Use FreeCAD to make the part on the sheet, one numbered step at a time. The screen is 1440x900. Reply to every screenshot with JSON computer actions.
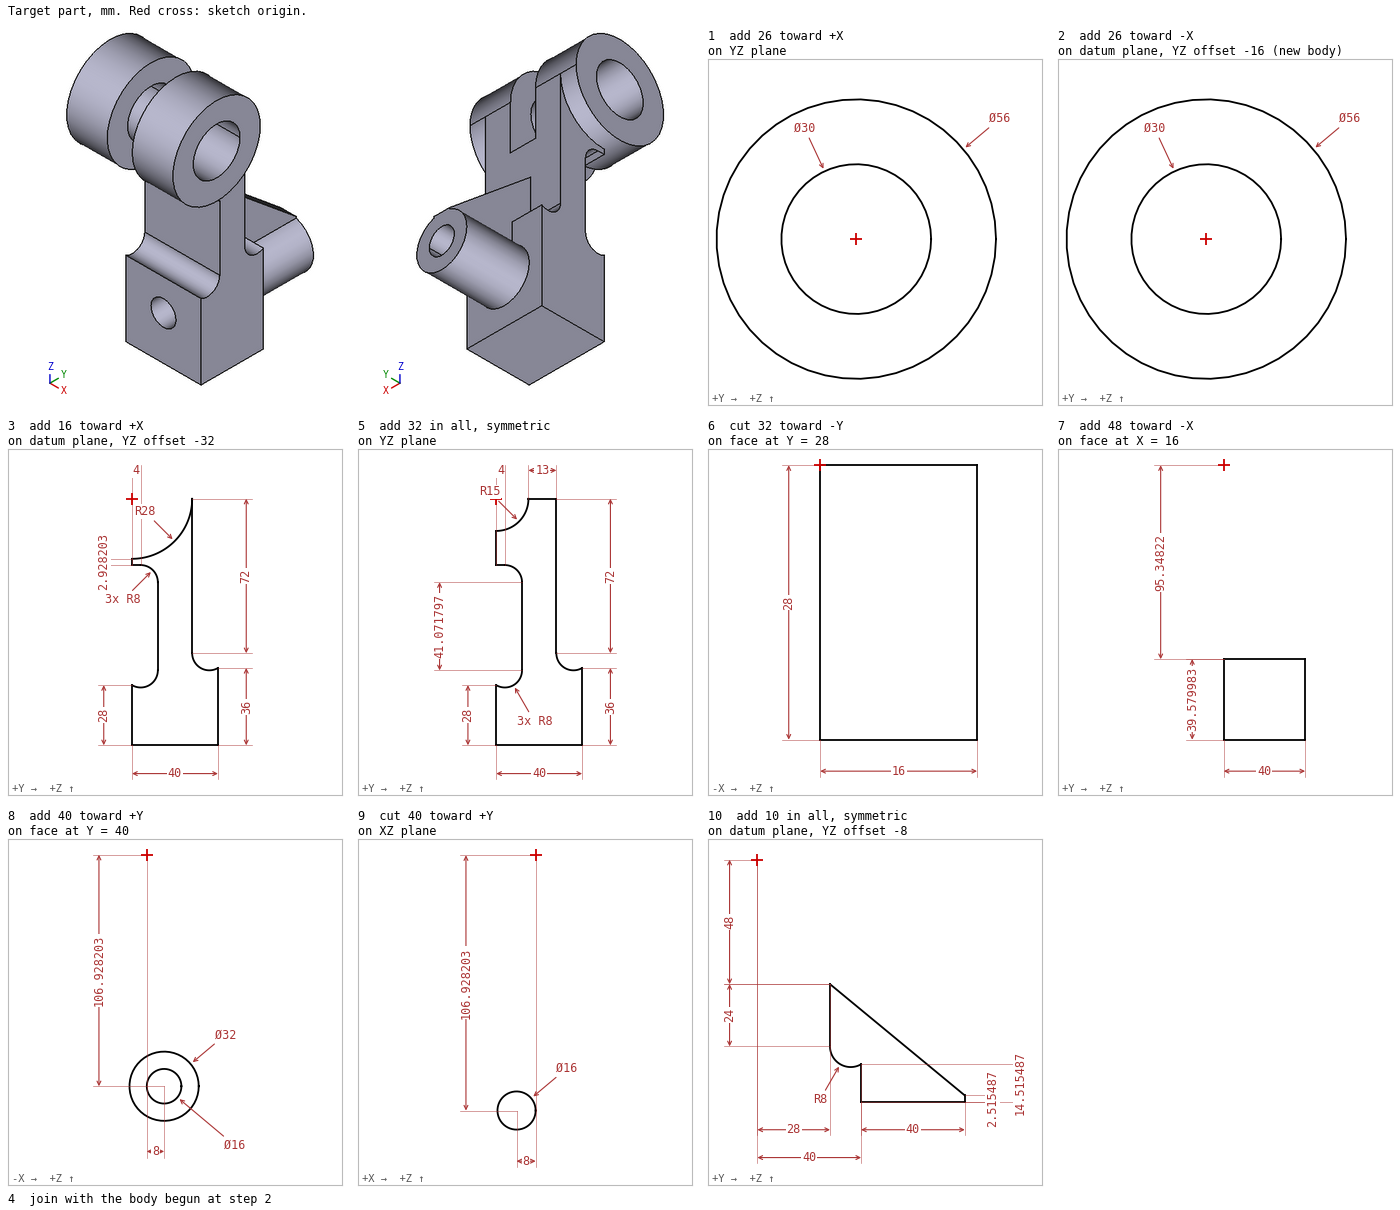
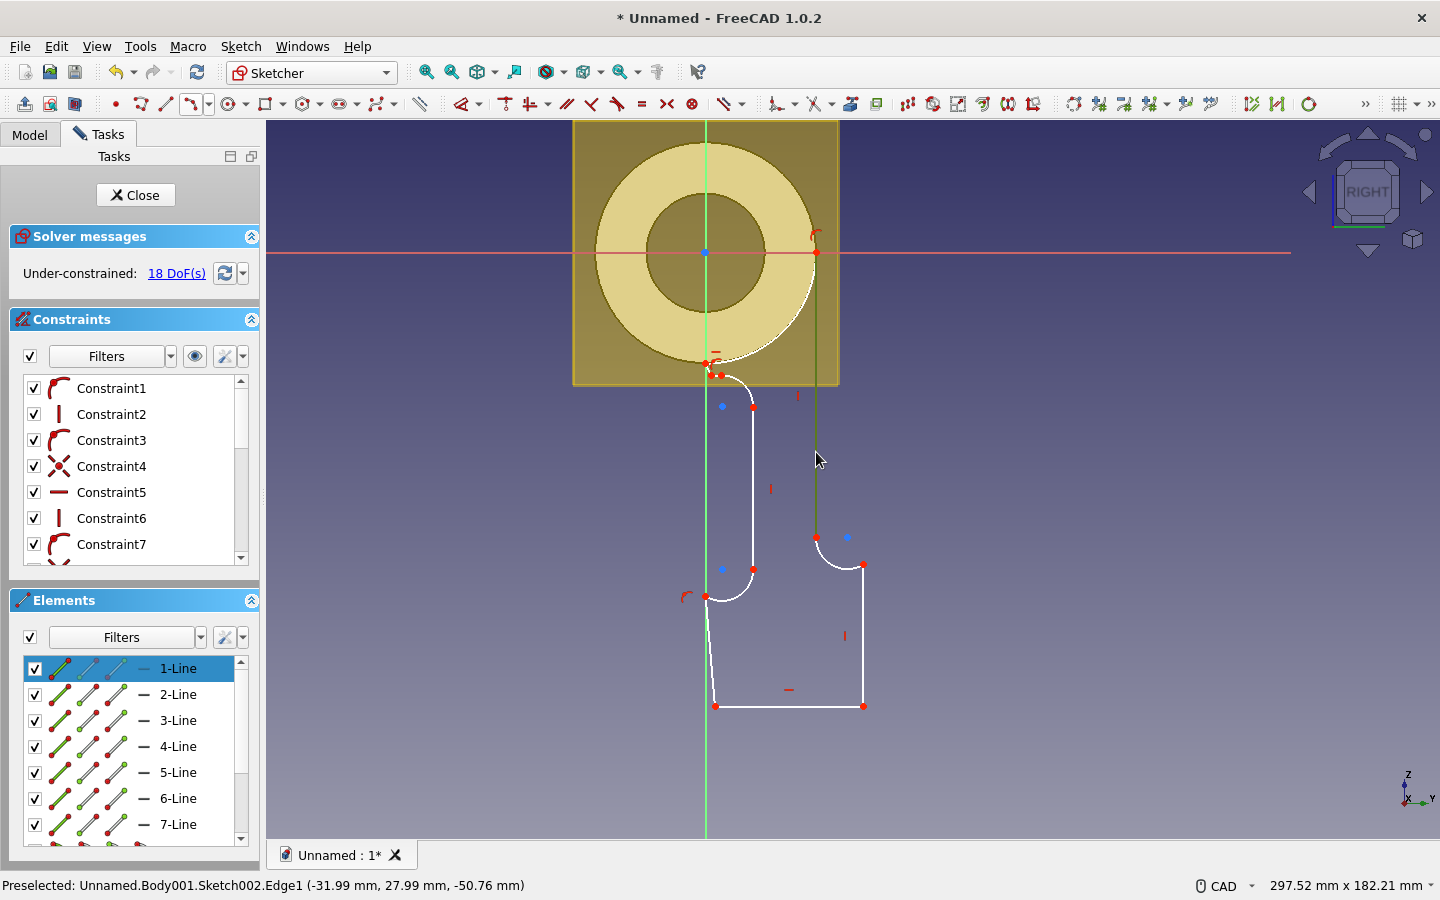
{"action": "left_click", "coordinate": [756, 351]}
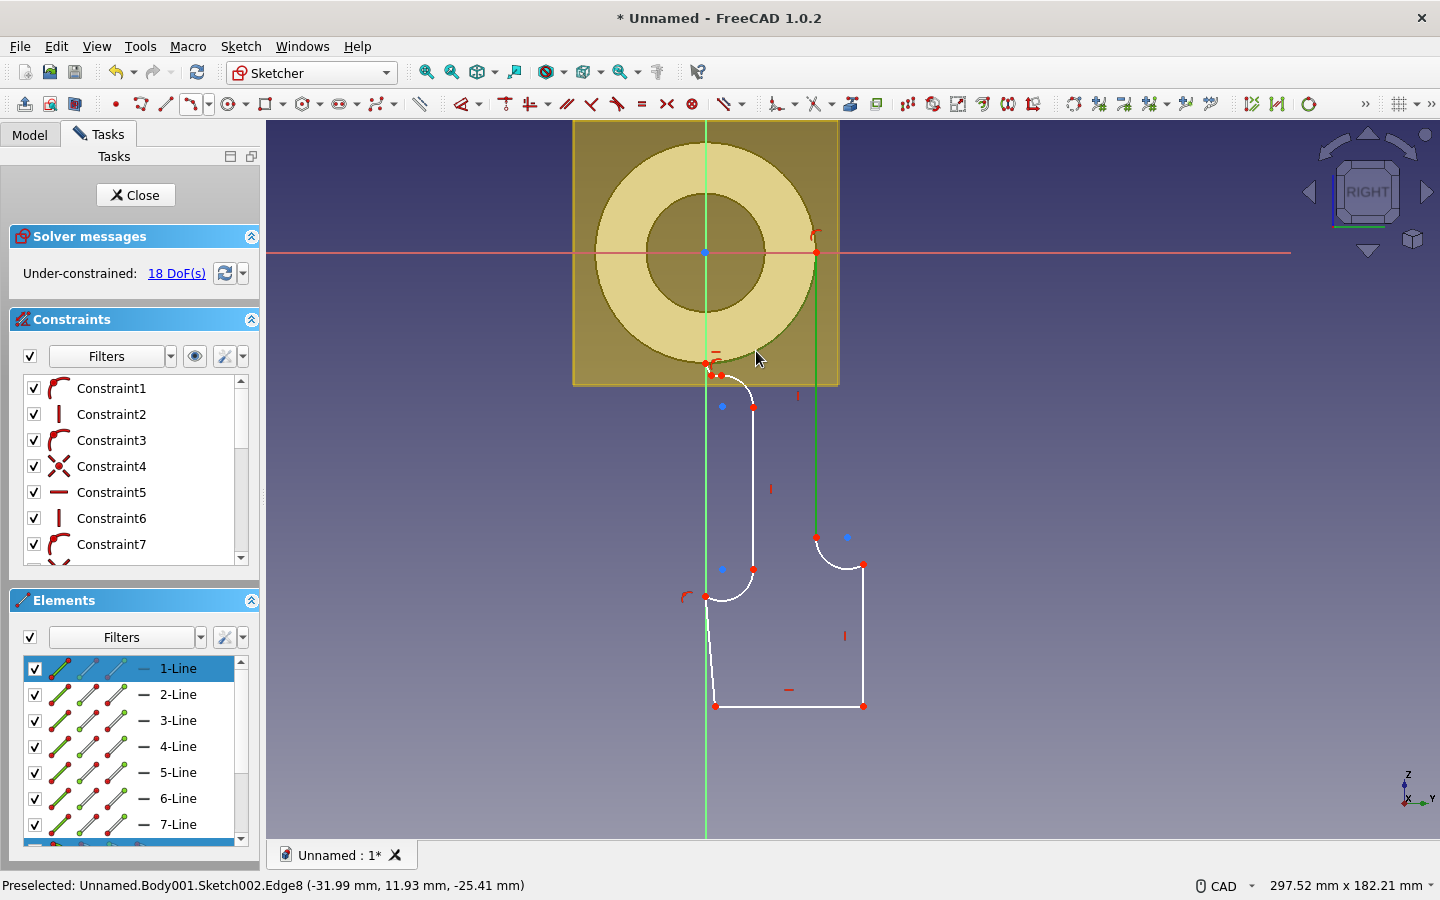
{"action": "key", "text": "t"}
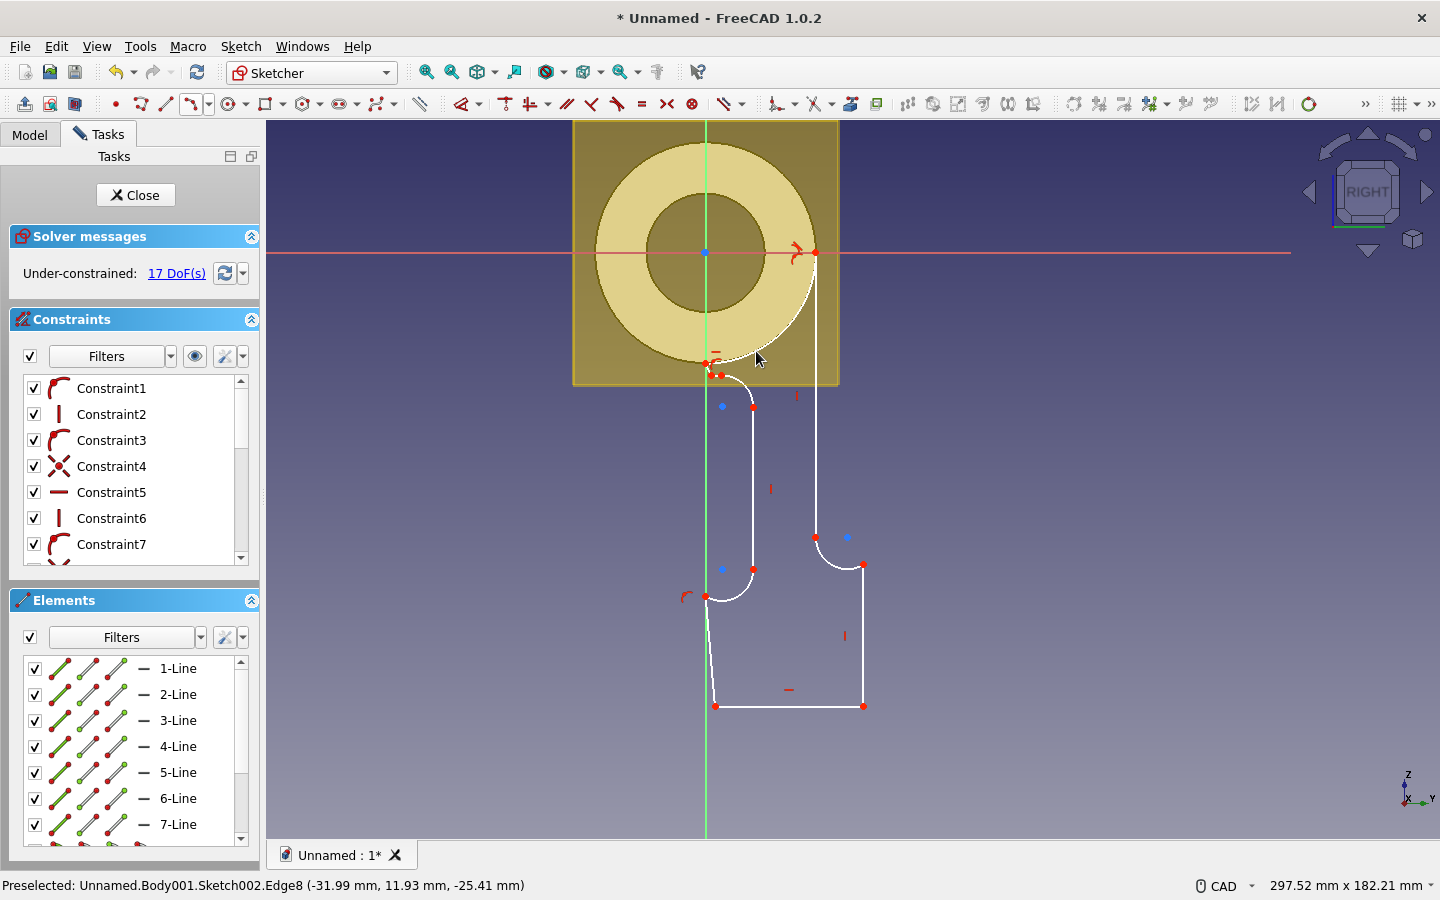
{"action": "left_click", "coordinate": [816, 452]}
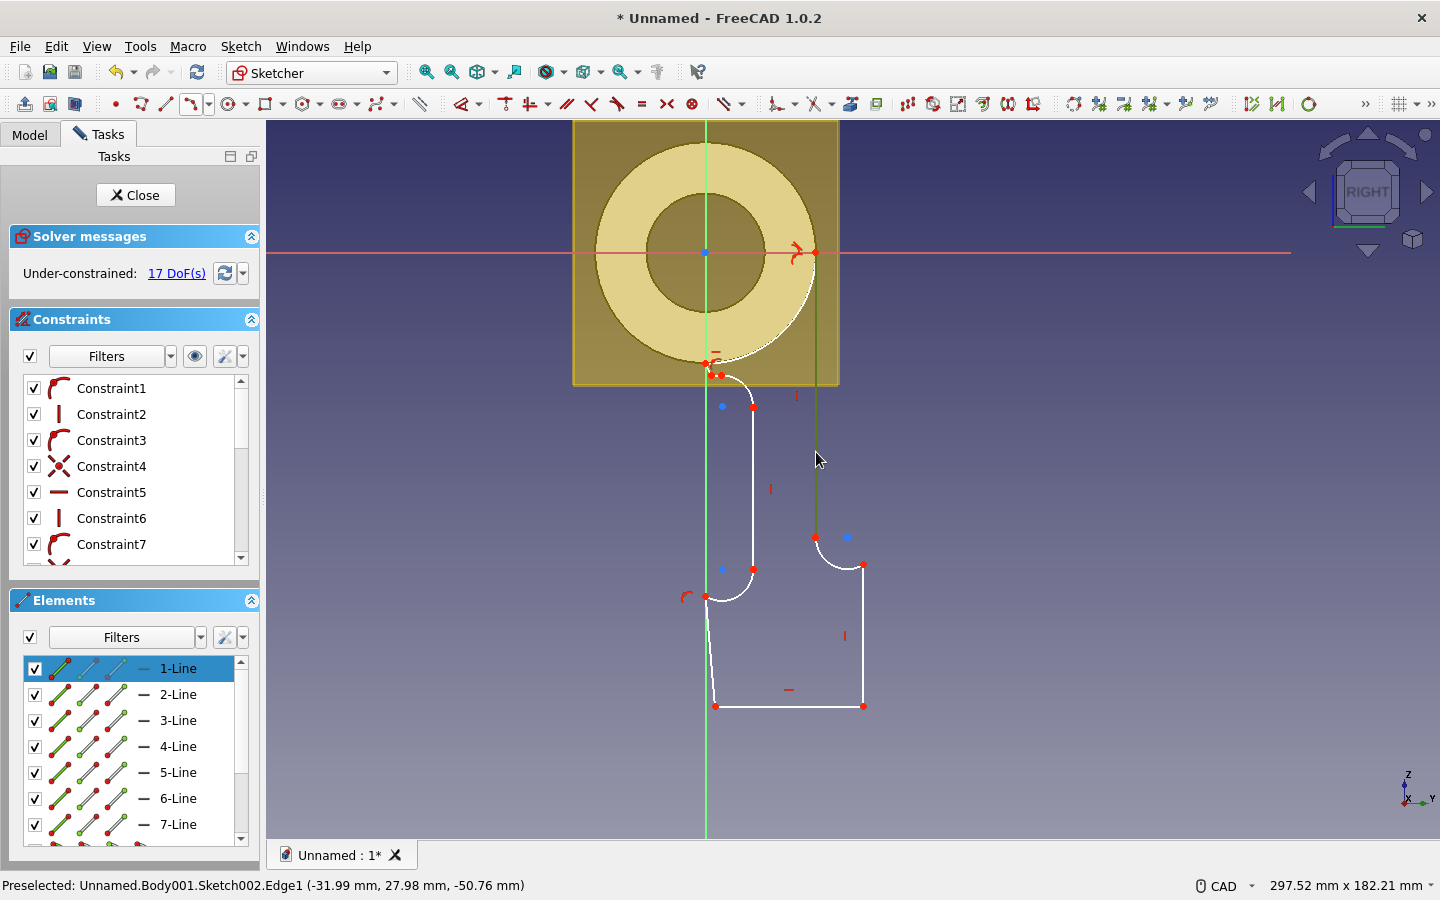
{"action": "left_click", "coordinate": [822, 556]}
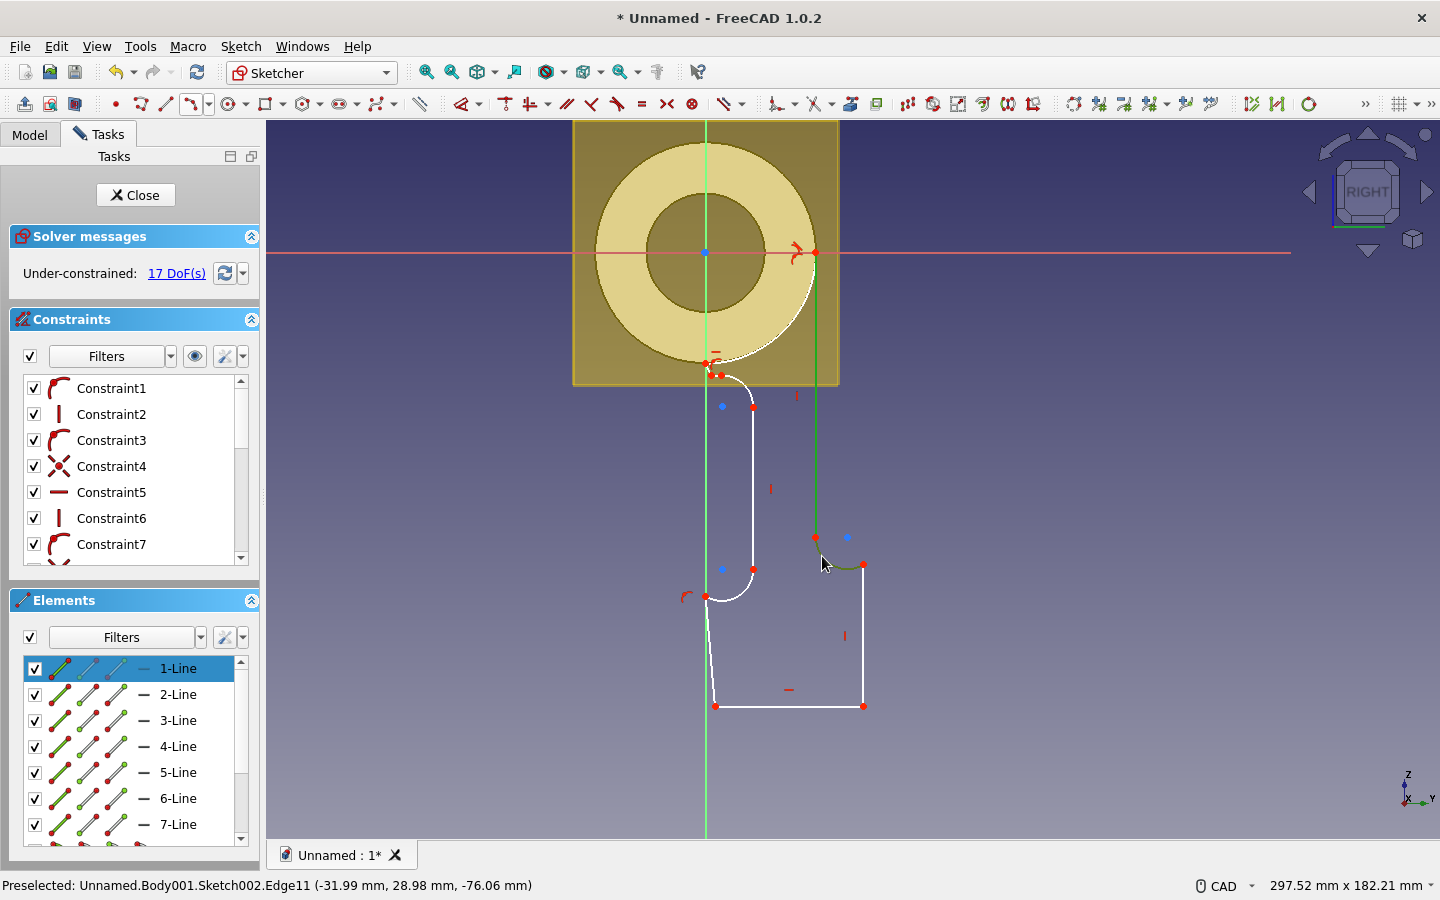
{"action": "key", "text": "t"}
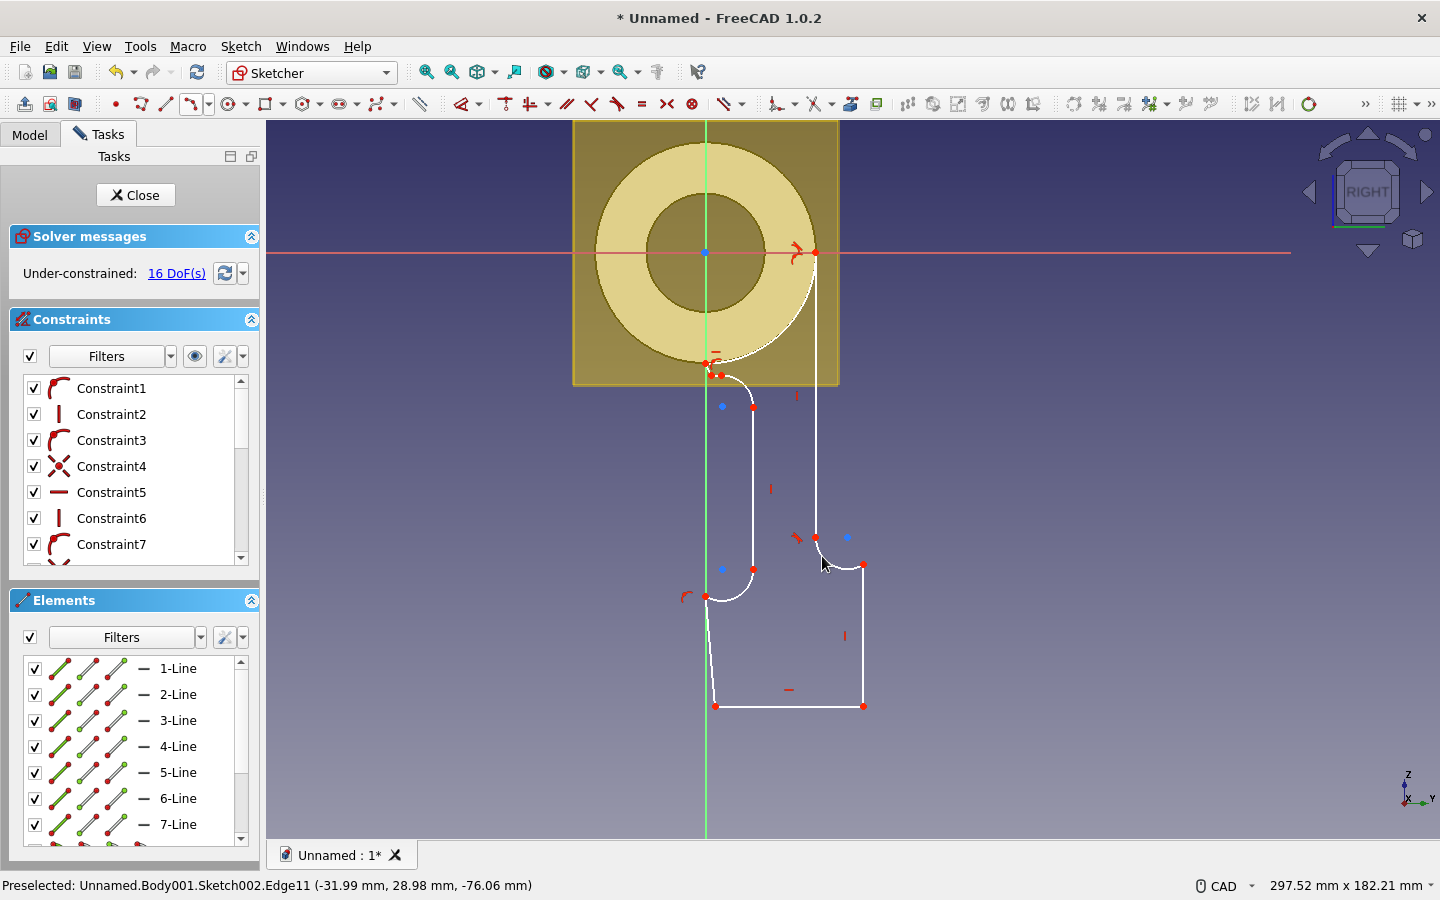
{"action": "scroll", "coordinate": [717, 376], "scroll_direction": "up", "scroll_amount": 6}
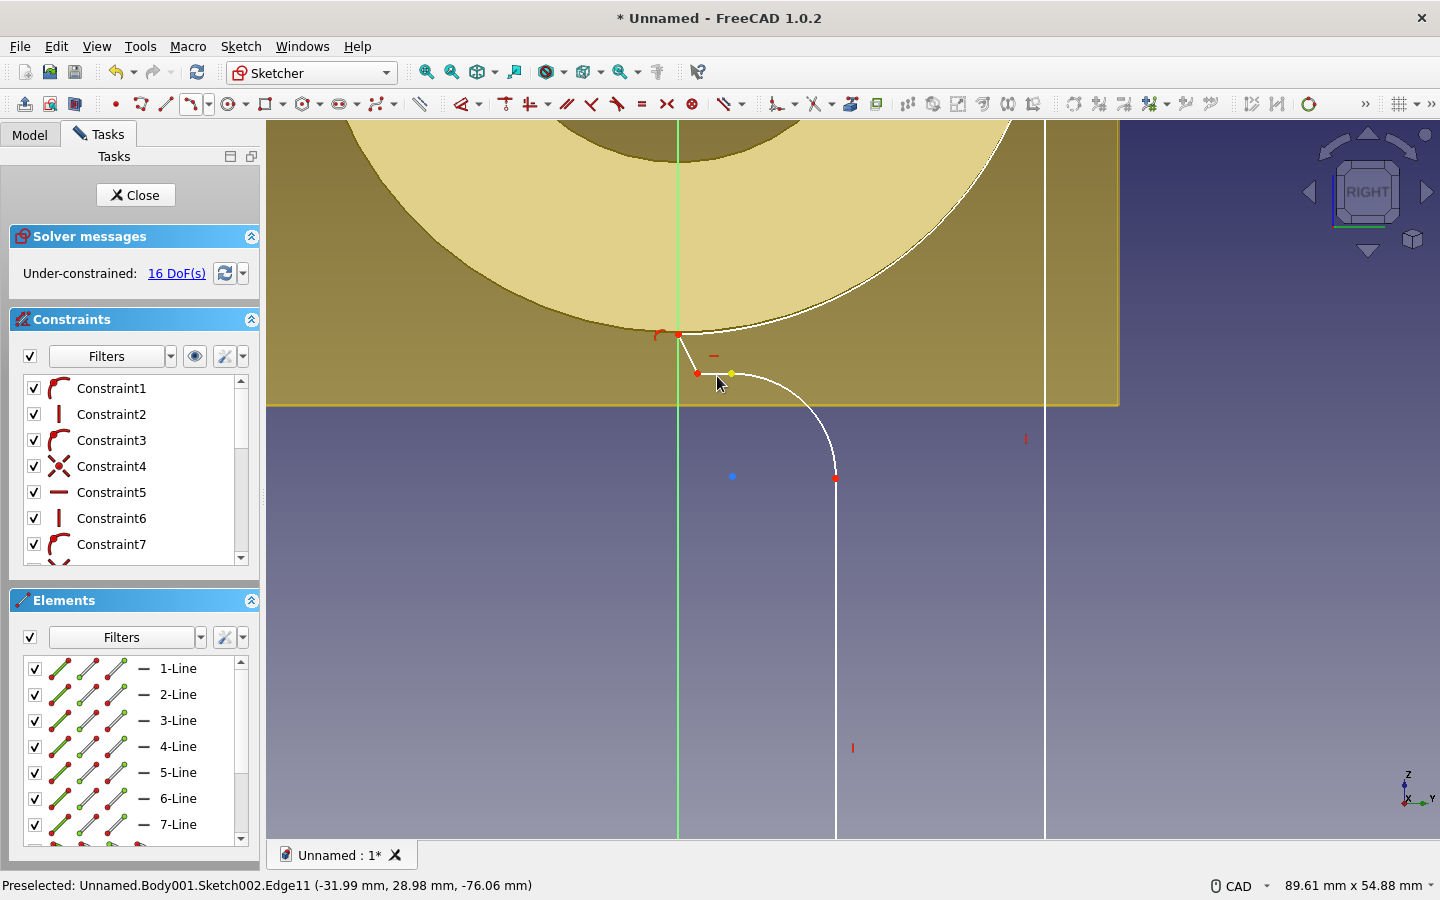
{"action": "left_click", "coordinate": [714, 374]}